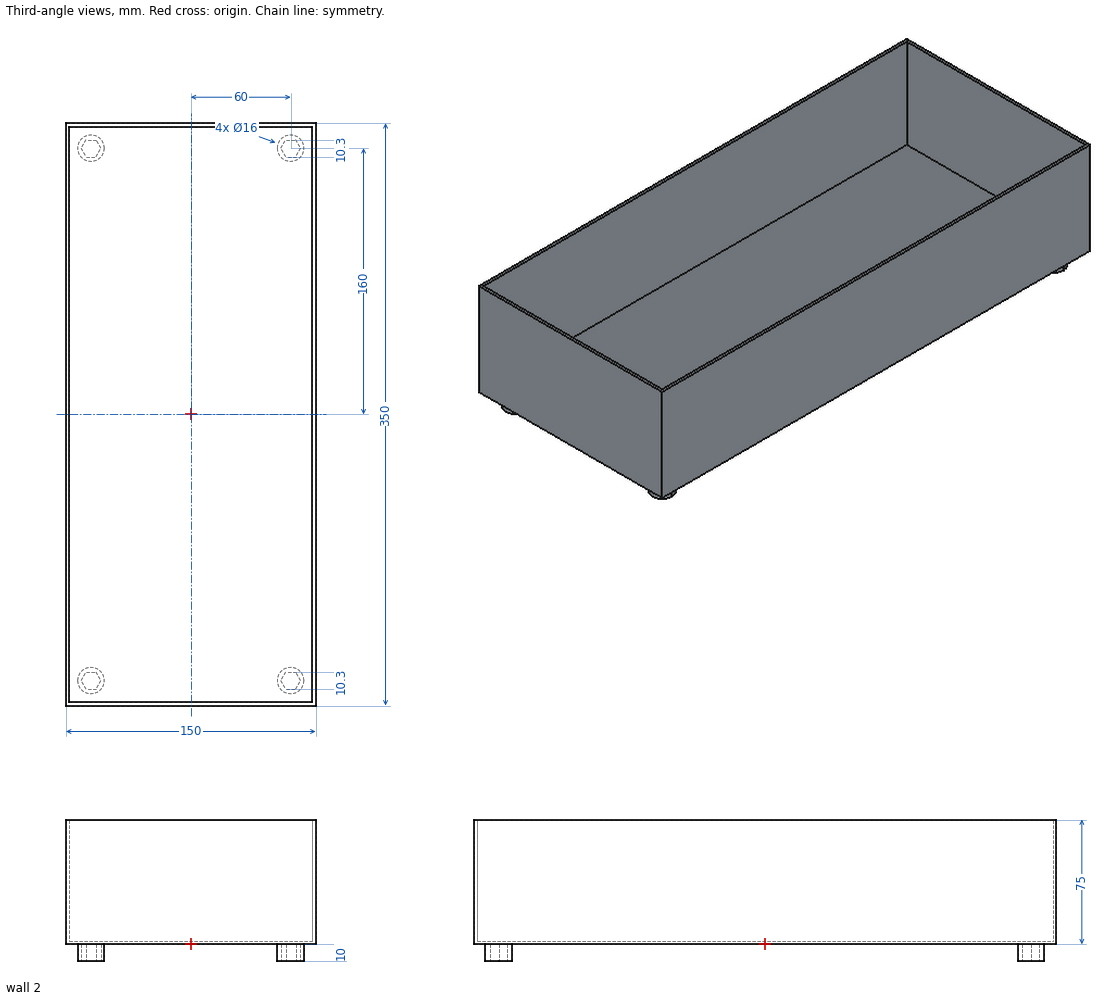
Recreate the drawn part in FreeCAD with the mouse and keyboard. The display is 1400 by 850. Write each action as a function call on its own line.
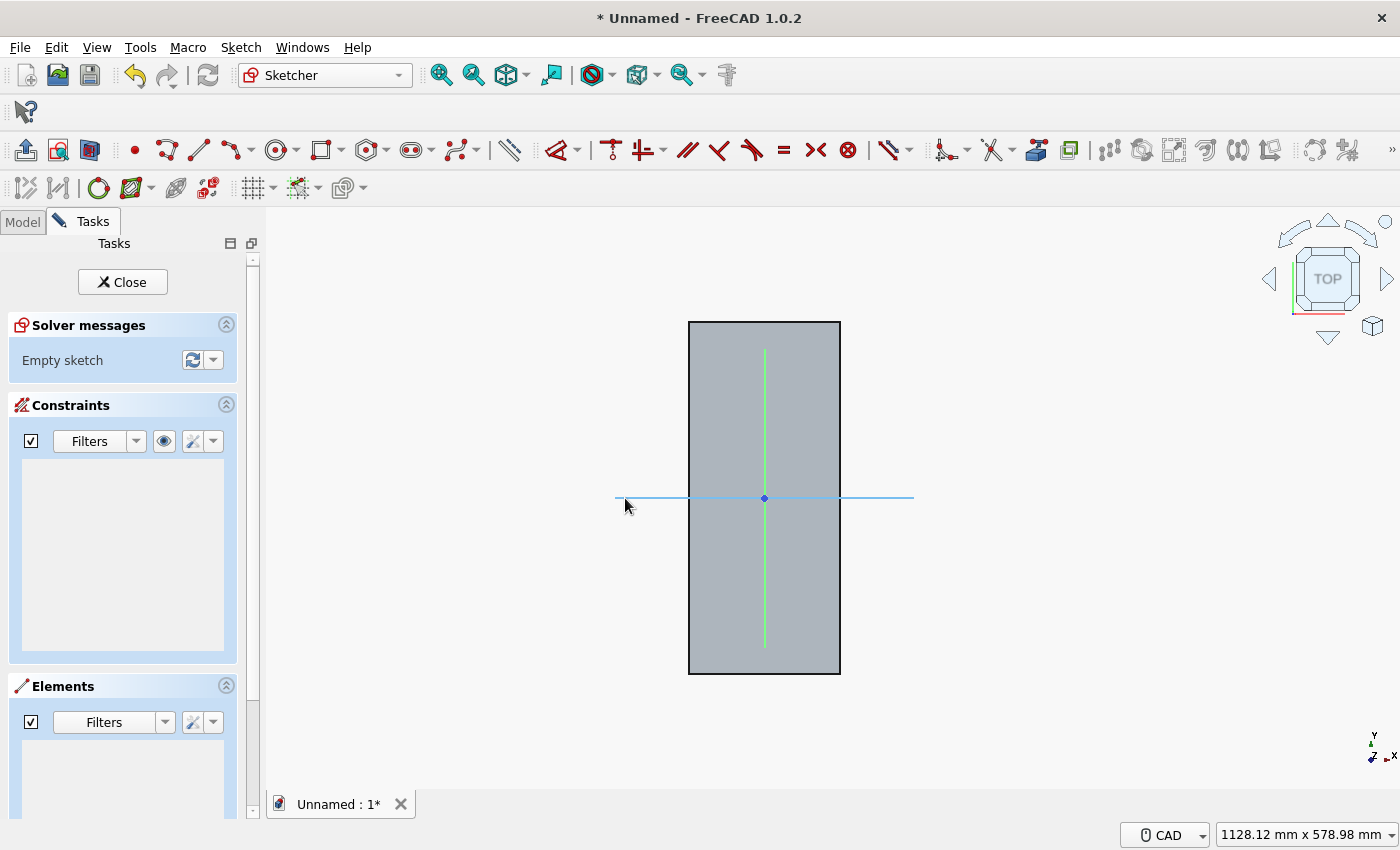
click(366, 150)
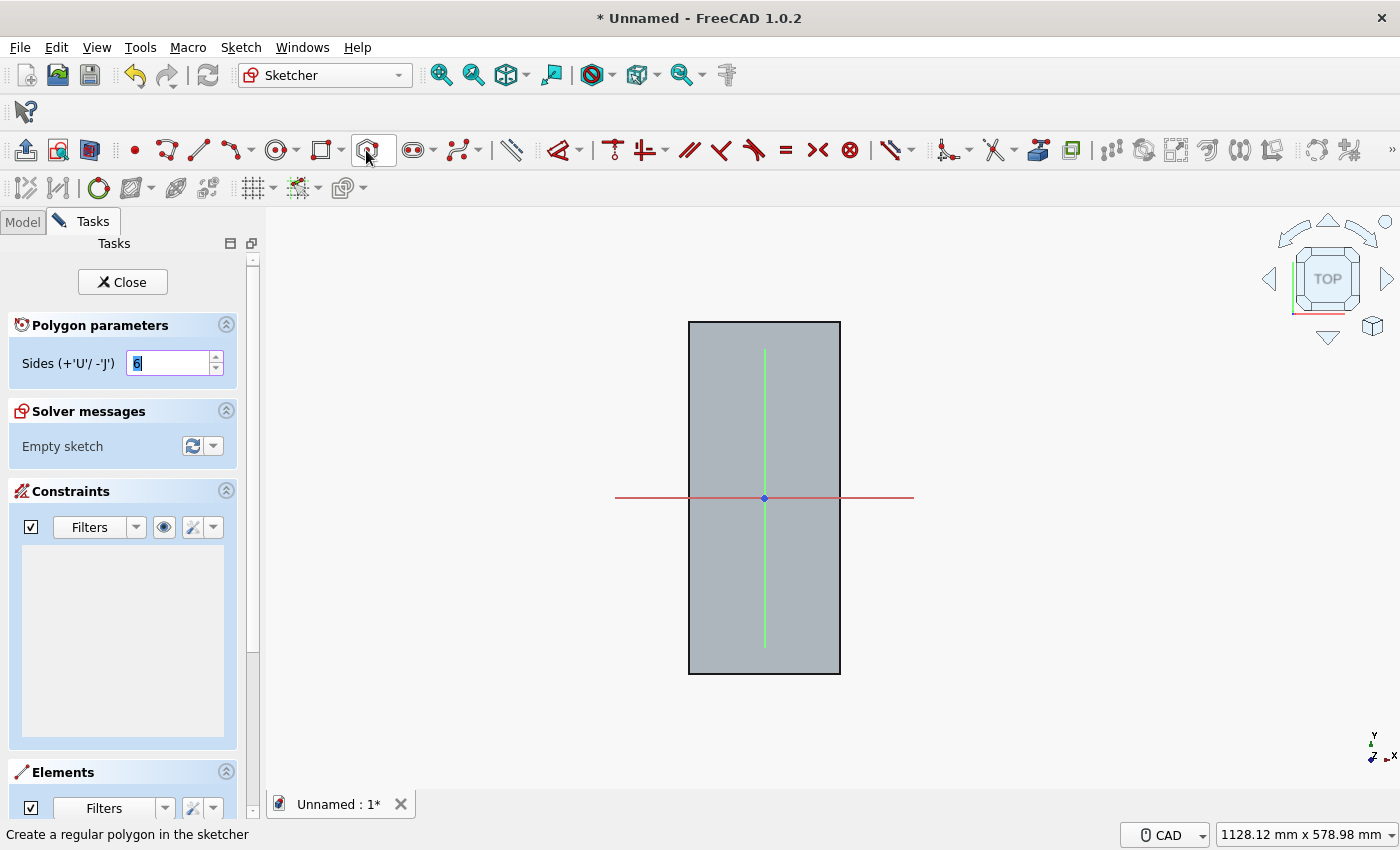
scroll(825, 337, up, 9)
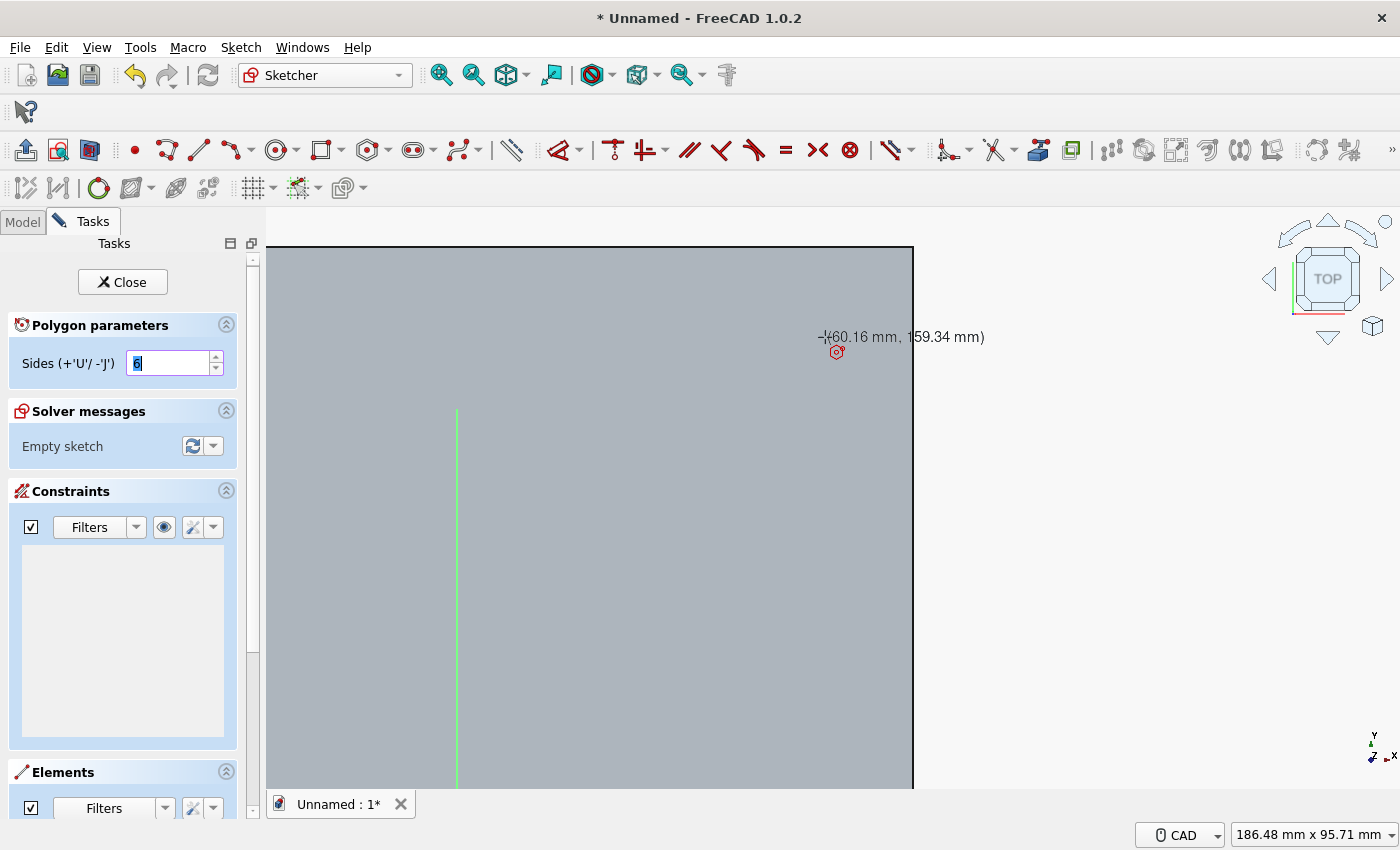
scroll(825, 337, down, 9)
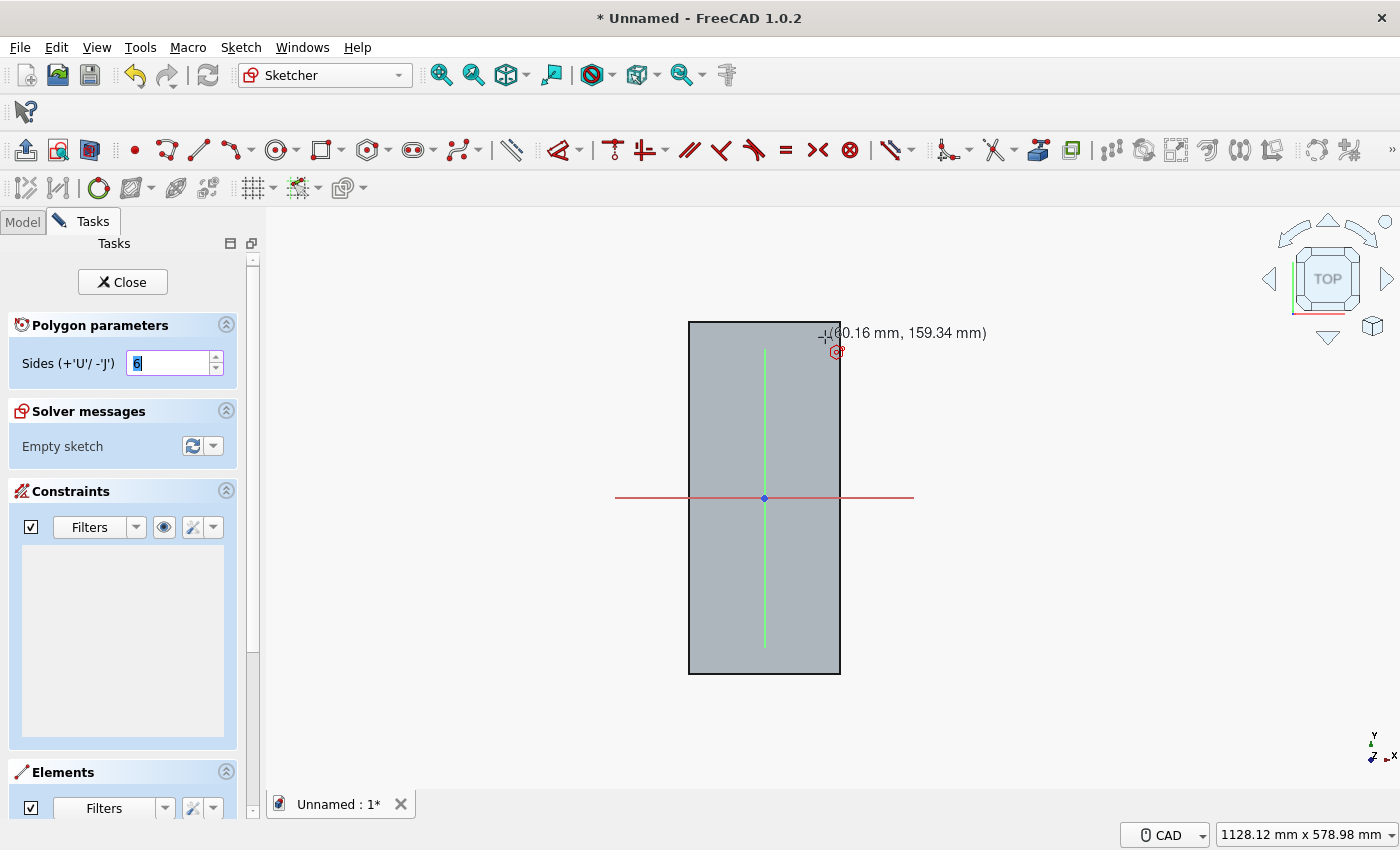
click(825, 337)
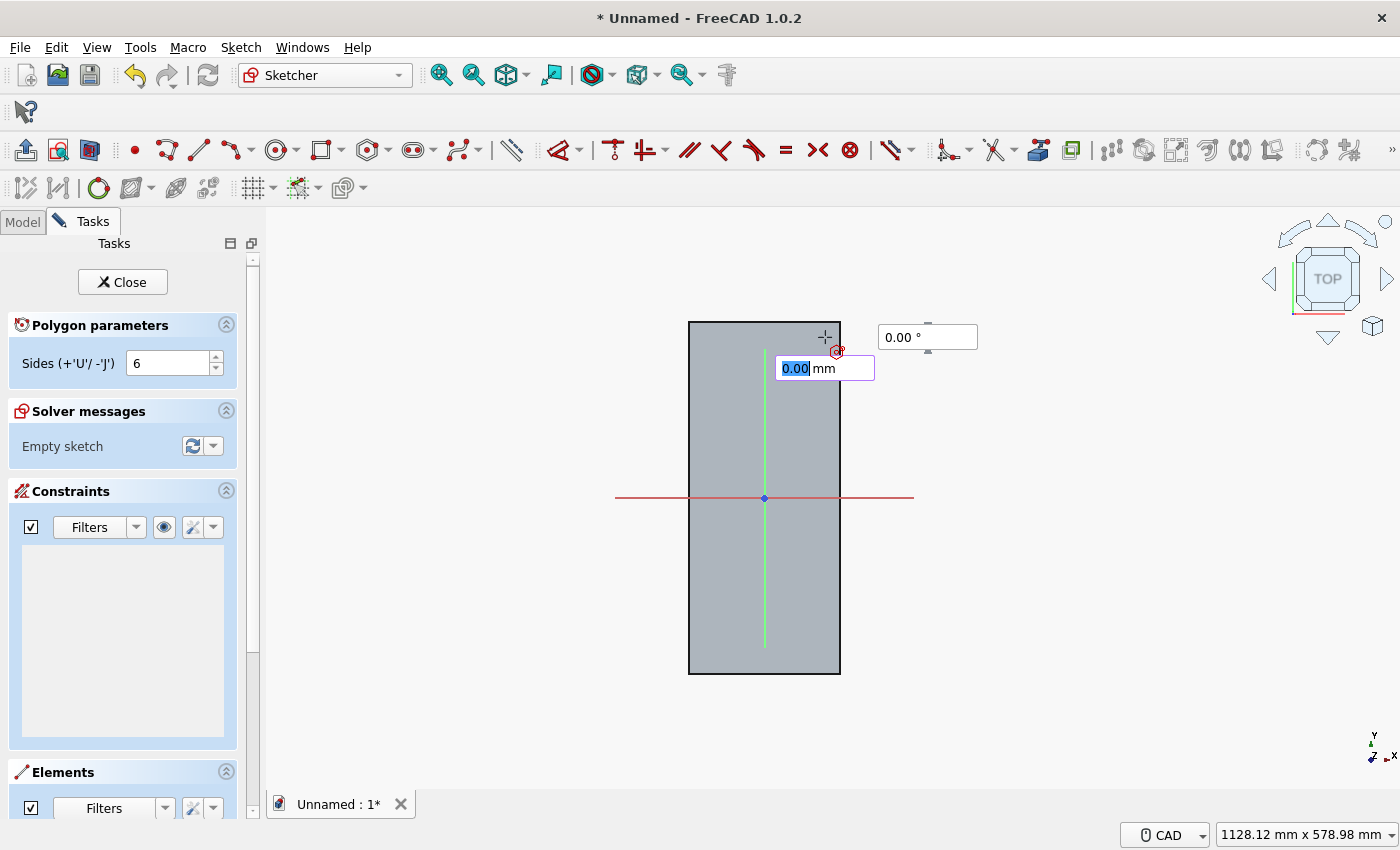
click(831, 337)
key(Escape)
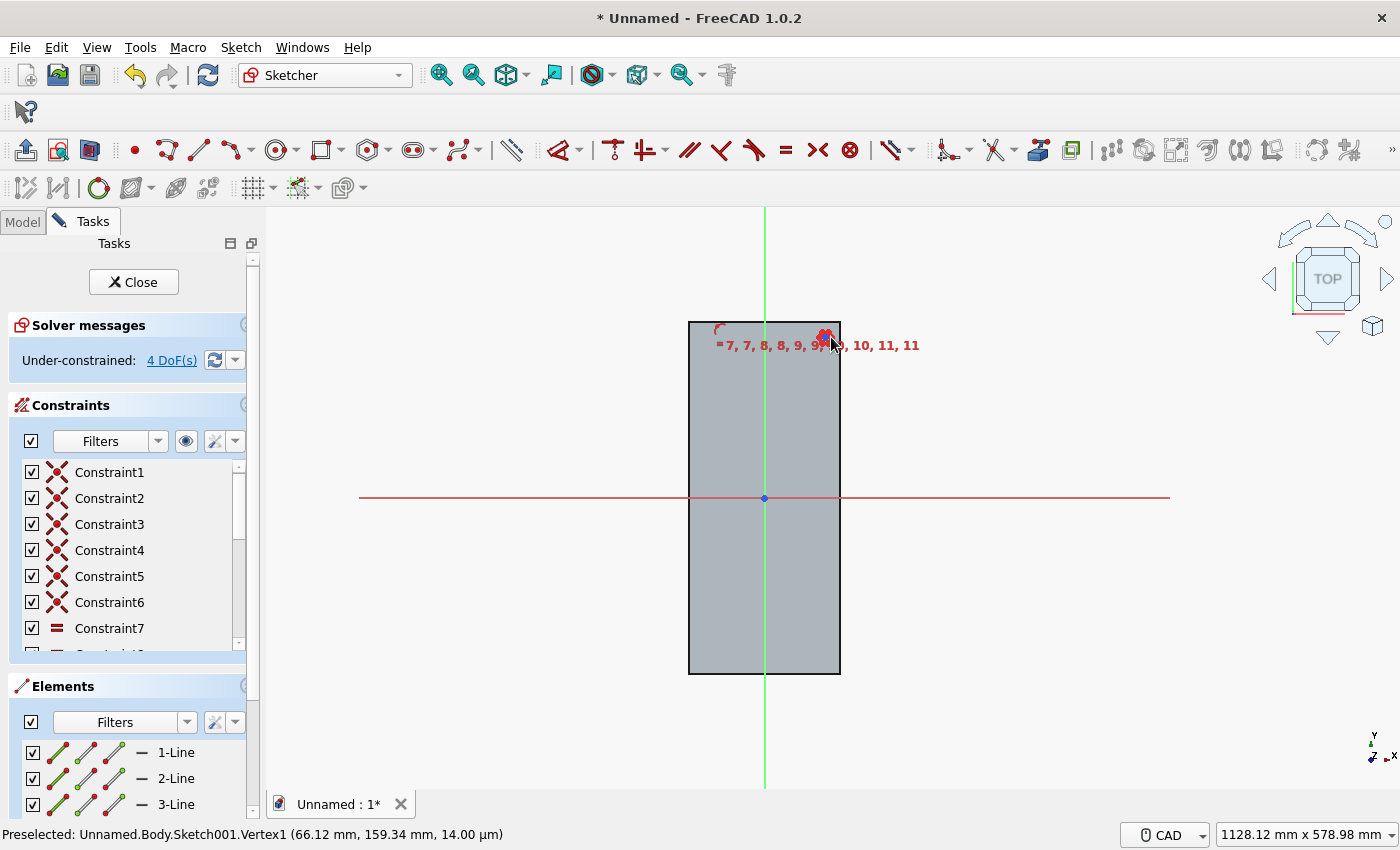
click(368, 150)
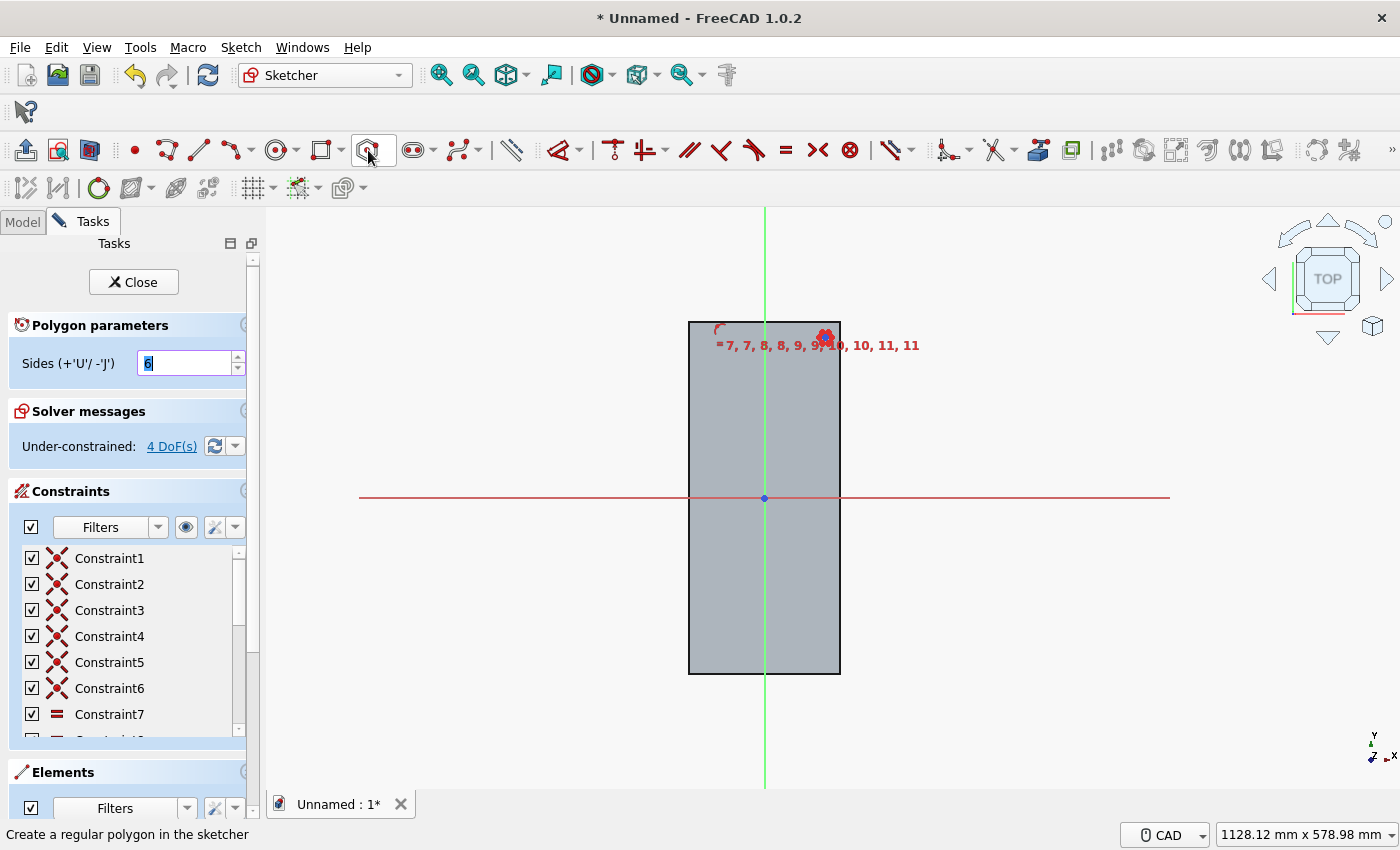
scroll(825, 659, up, 9)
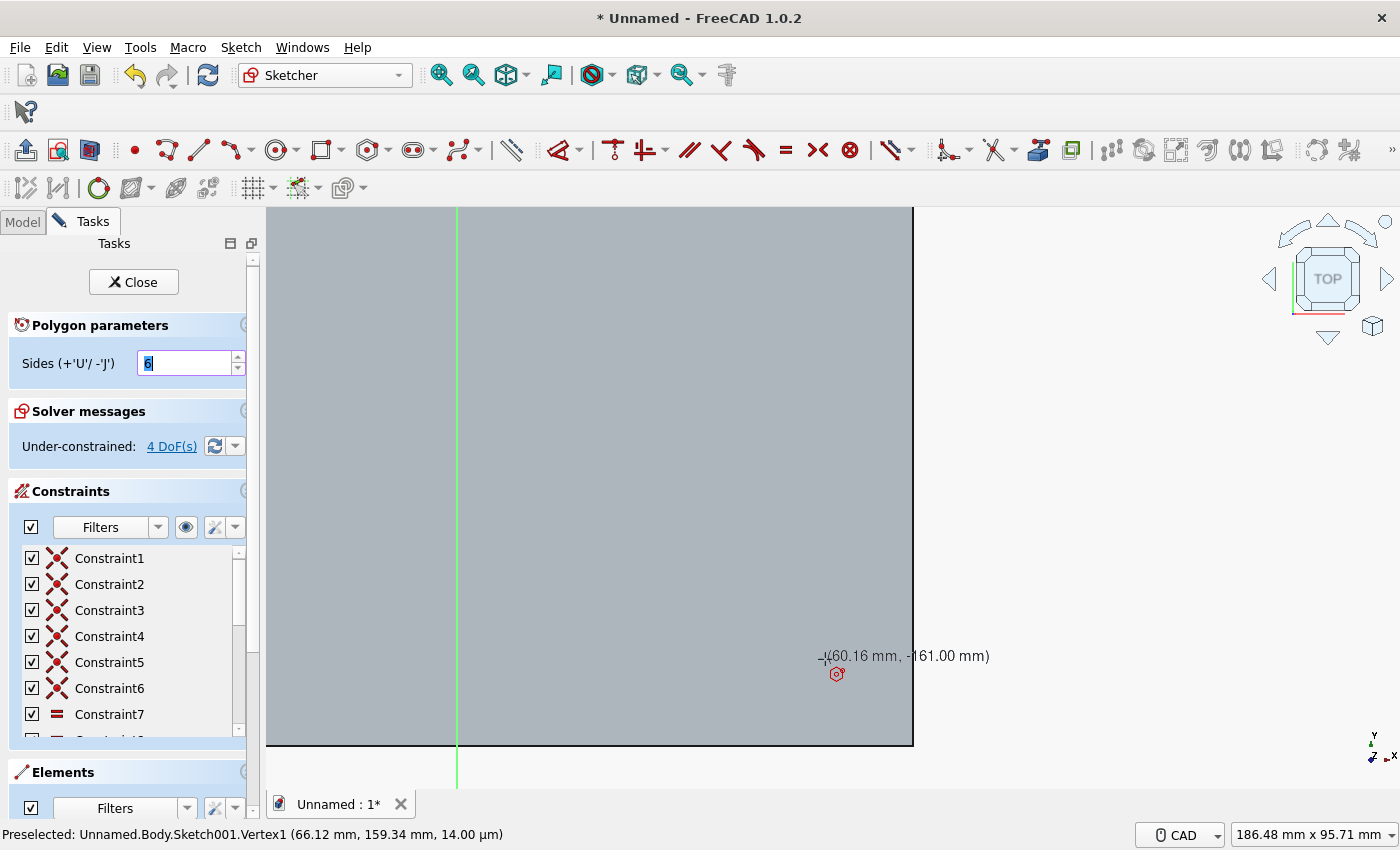
scroll(825, 660, down, 9)